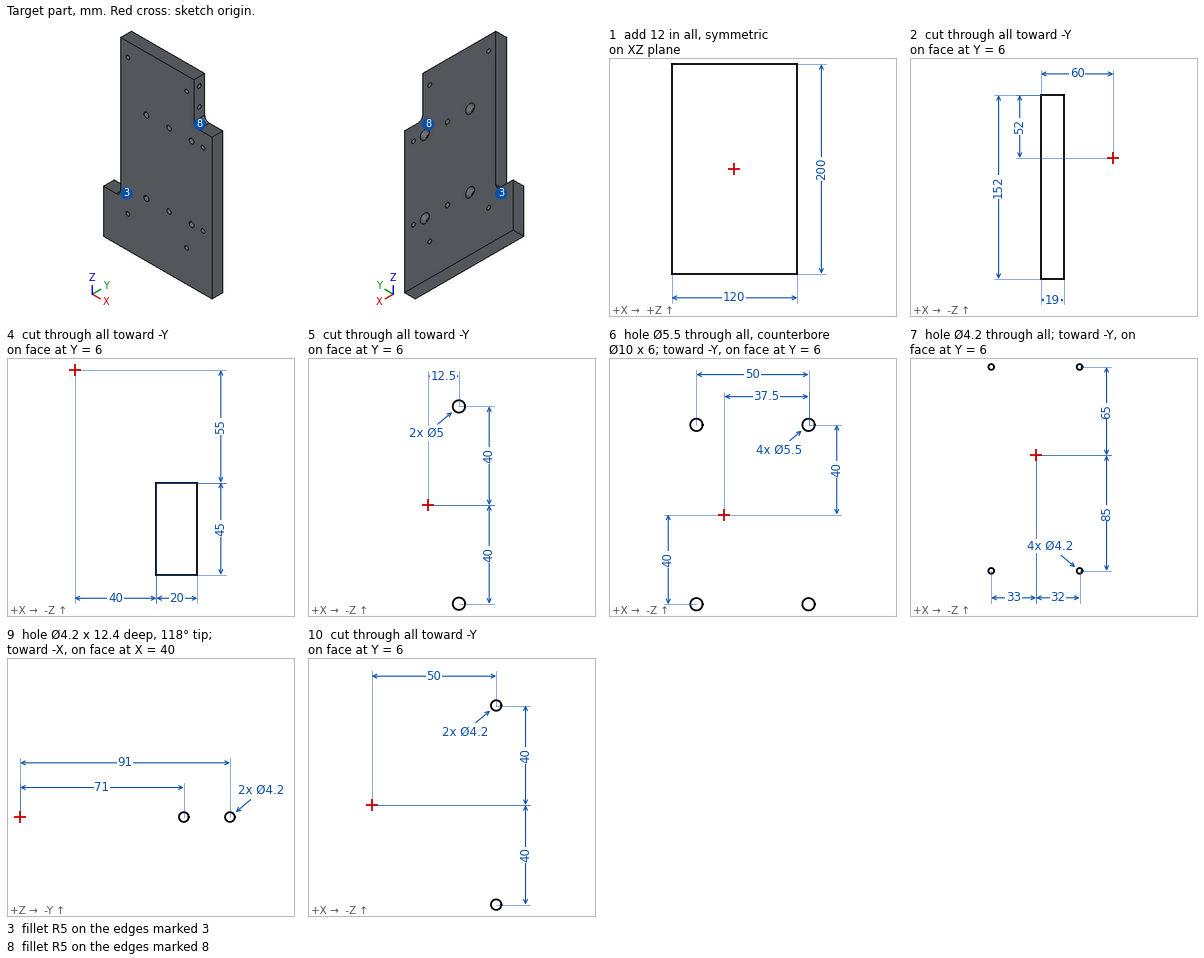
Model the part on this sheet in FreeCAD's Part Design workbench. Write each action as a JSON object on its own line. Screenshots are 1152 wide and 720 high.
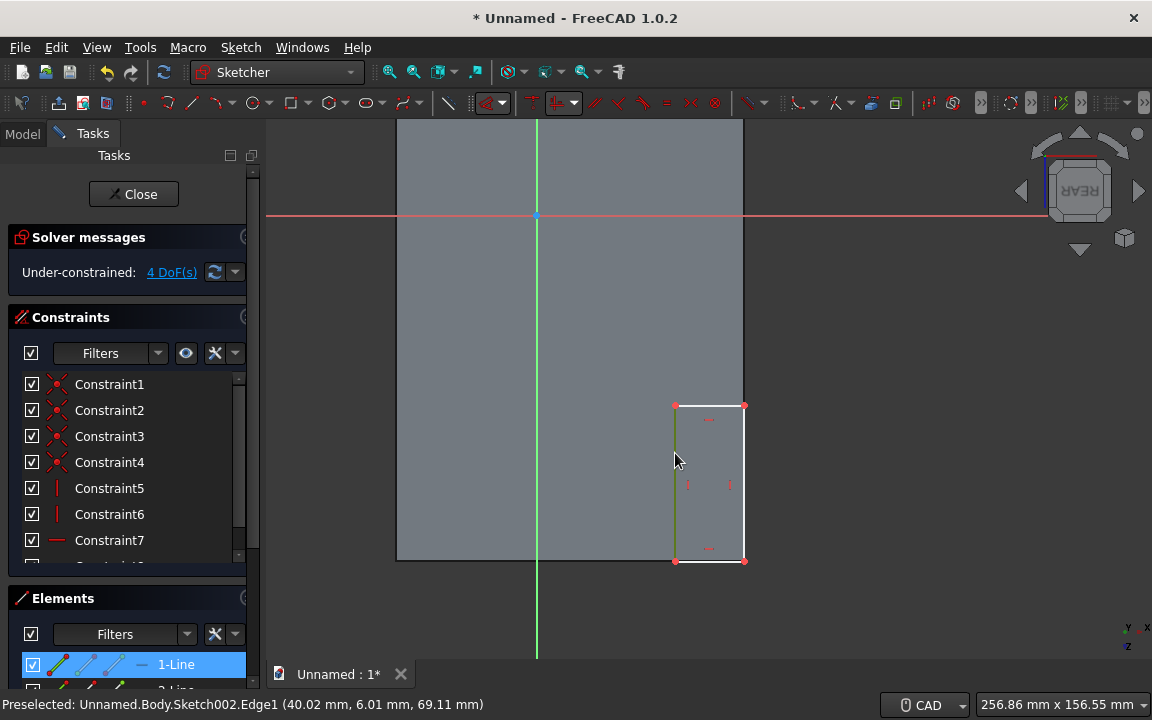
{"action": "left_click", "coordinate": [504, 104]}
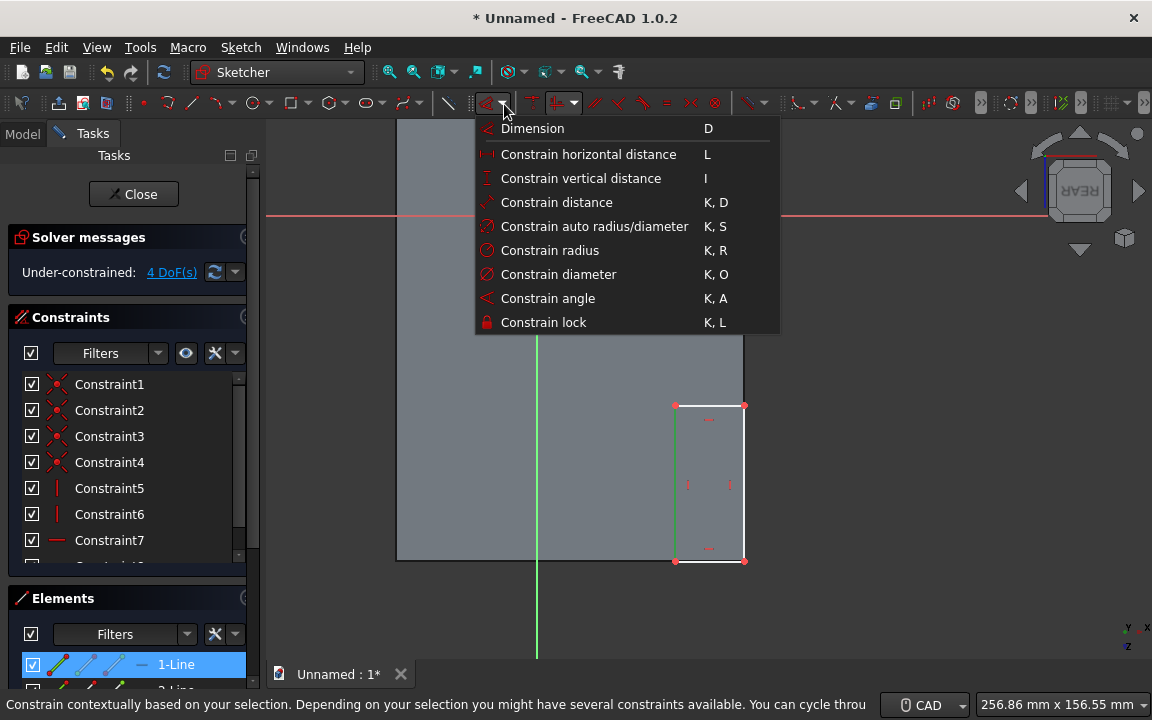
{"action": "left_click", "coordinate": [628, 178]}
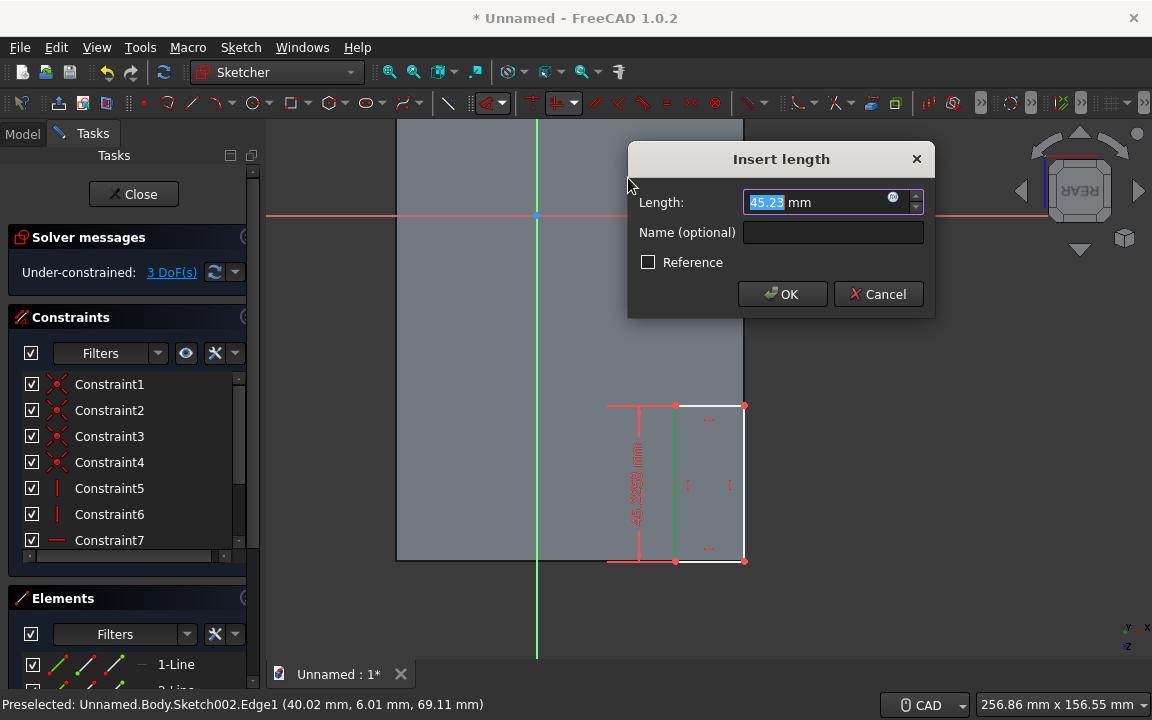
{"action": "type", "text": "45"}
{"action": "key", "text": "Return"}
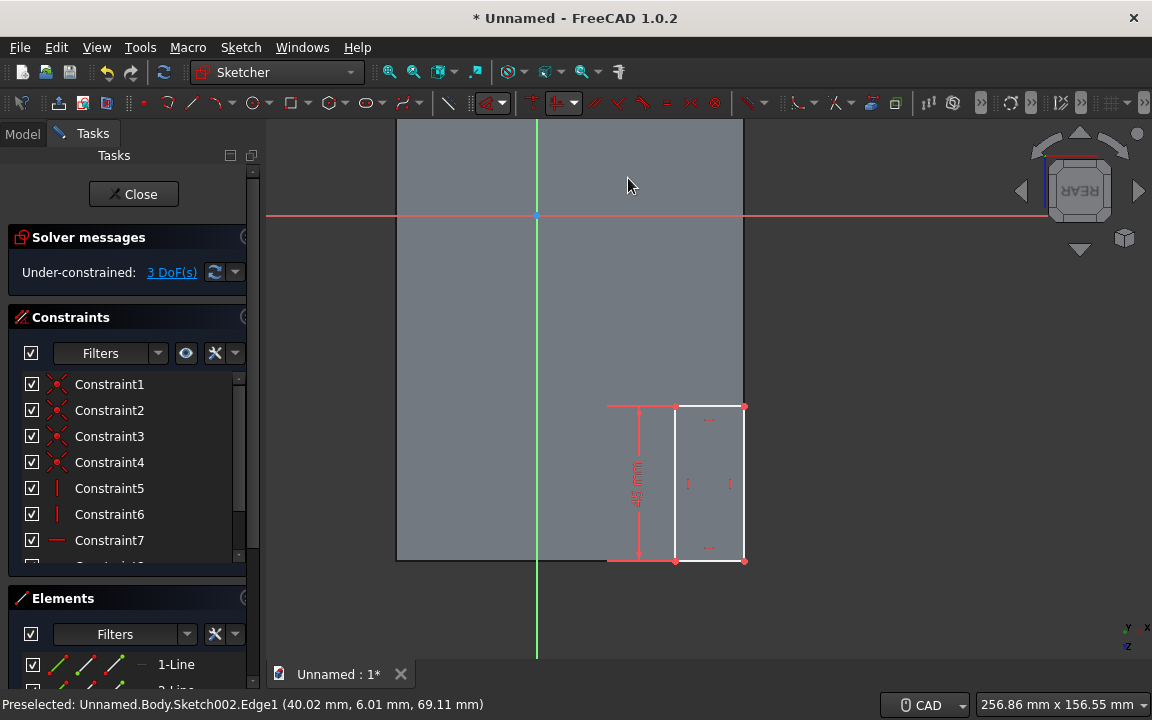
{"action": "left_click", "coordinate": [696, 561]}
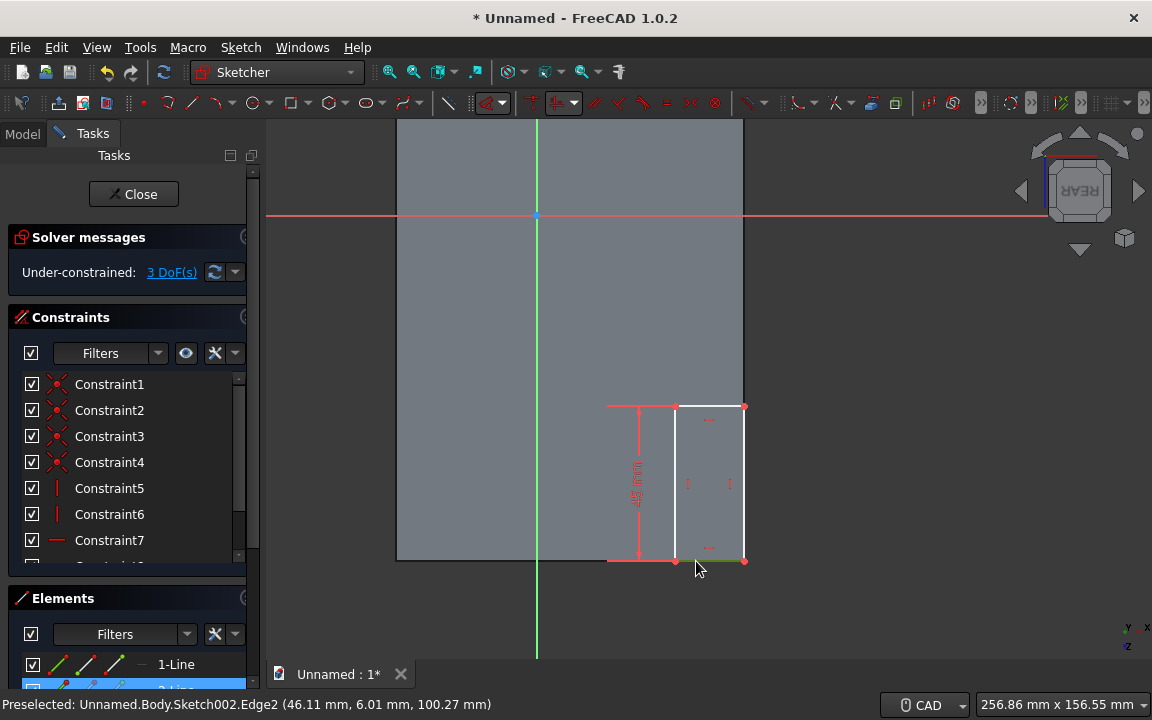
{"action": "left_click", "coordinate": [504, 104]}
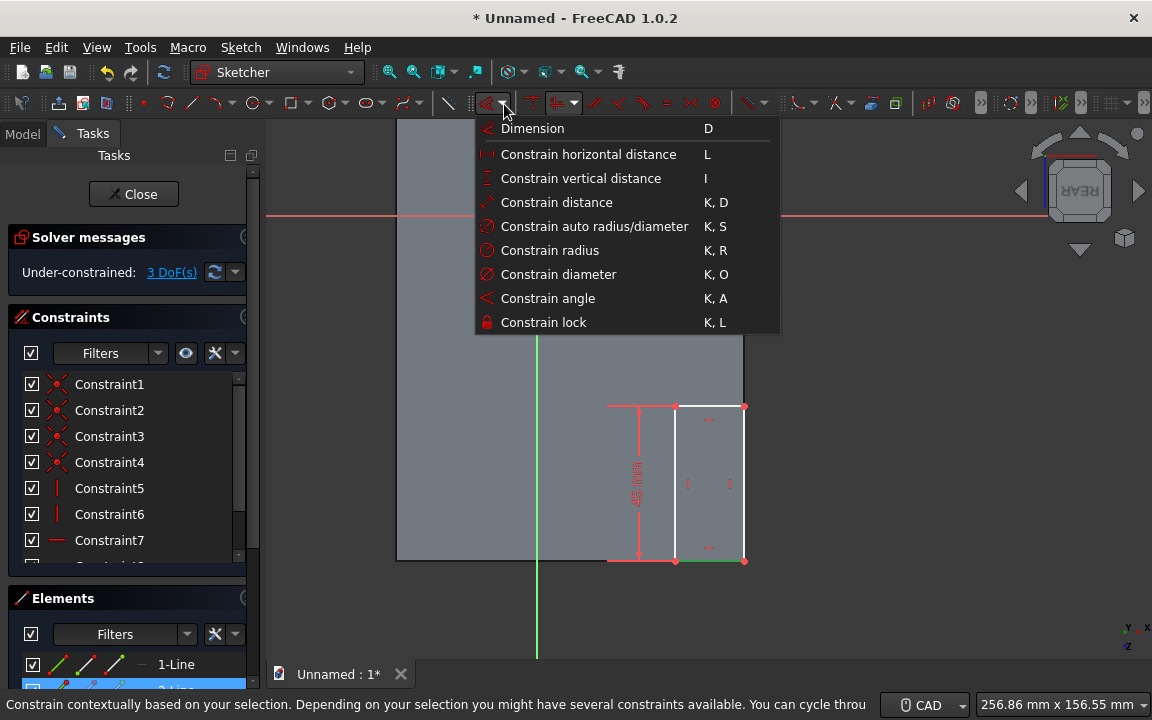
{"action": "left_click", "coordinate": [628, 154]}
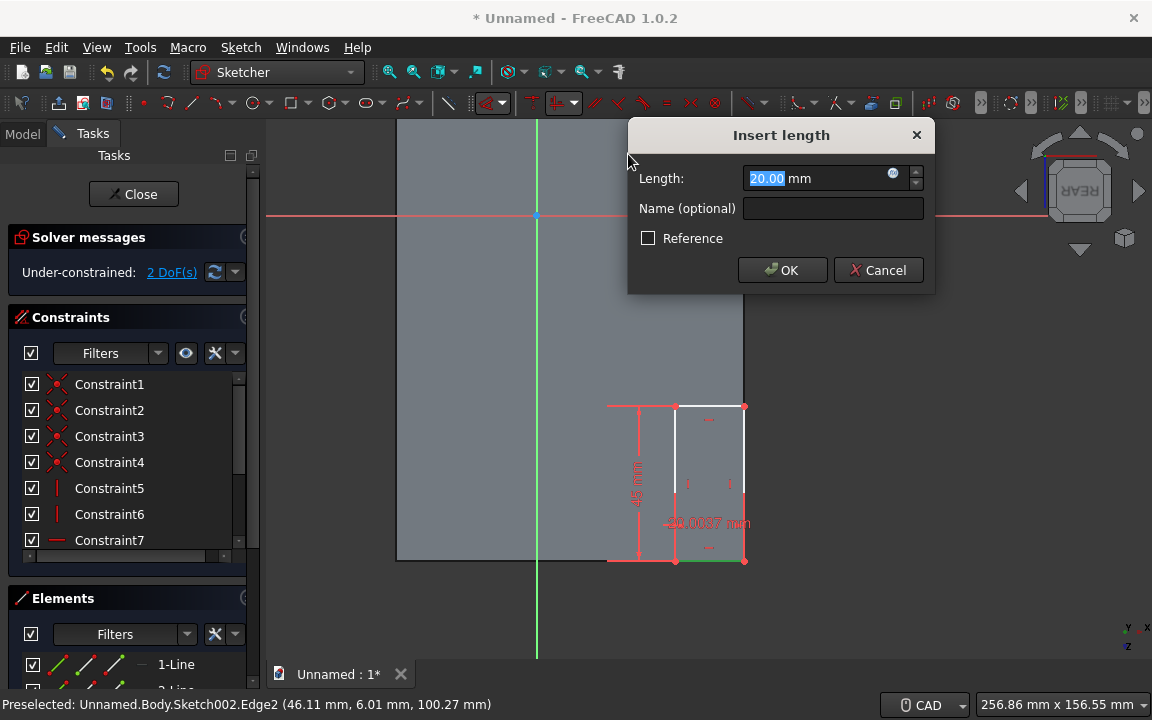
{"action": "type", "text": "20"}
{"action": "key", "text": "Return"}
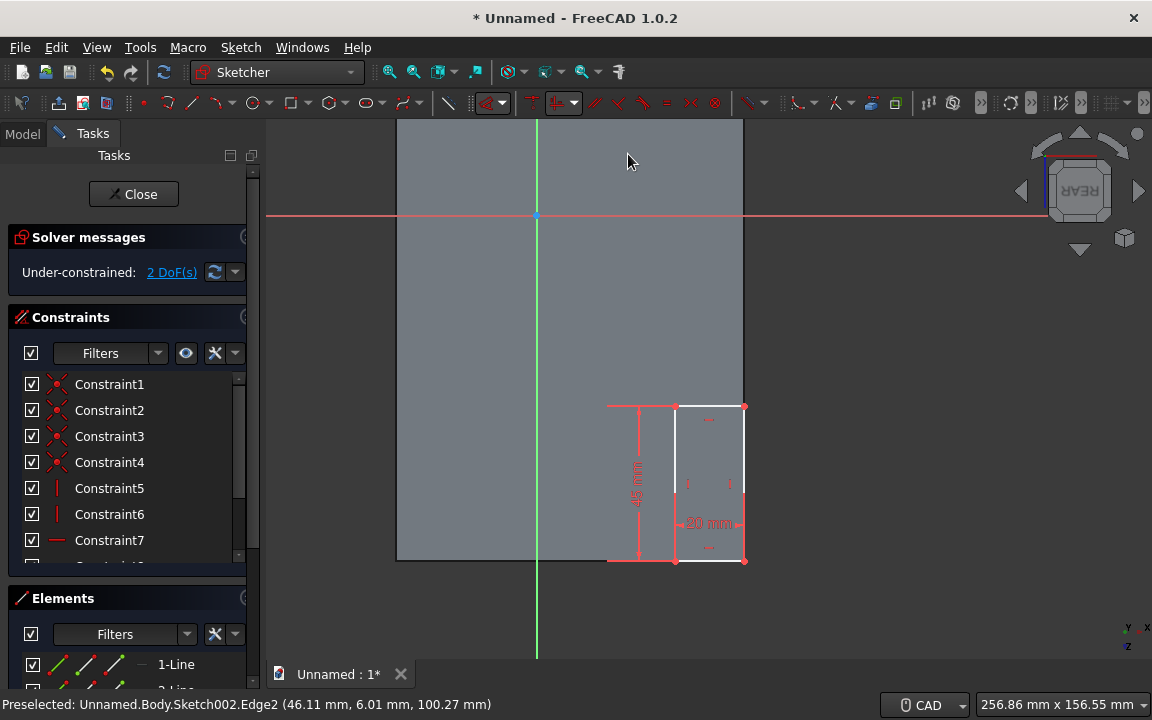
{"action": "left_click", "coordinate": [675, 406]}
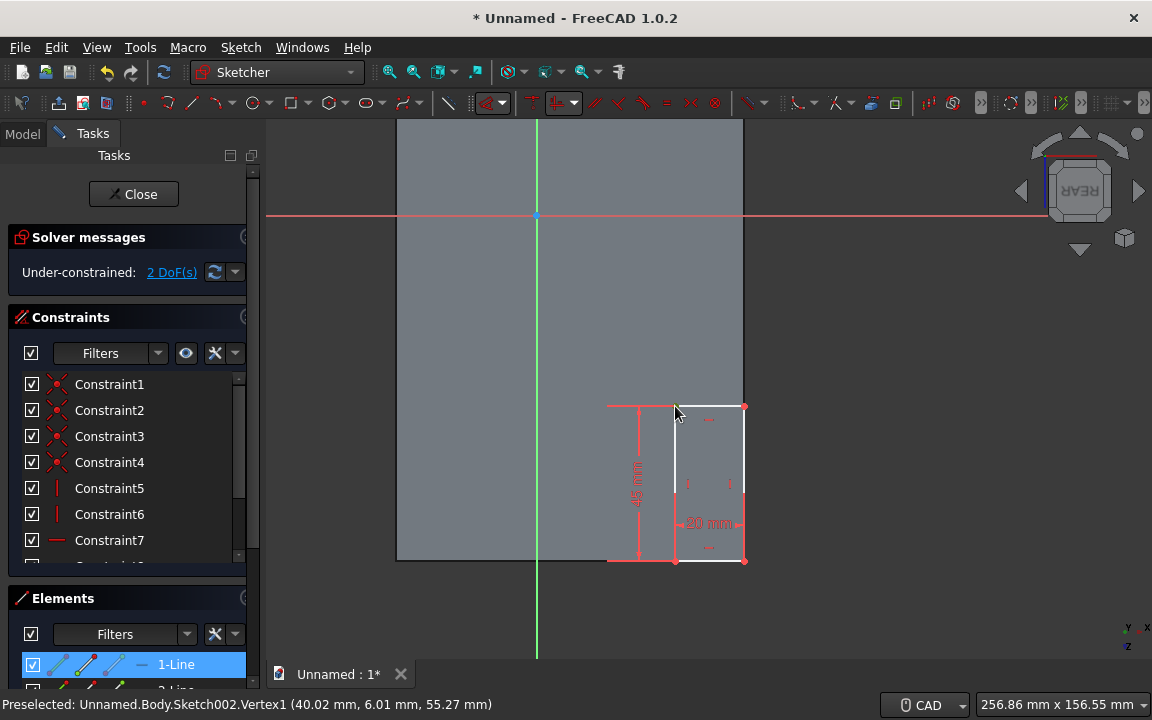
{"action": "key", "text": "l"}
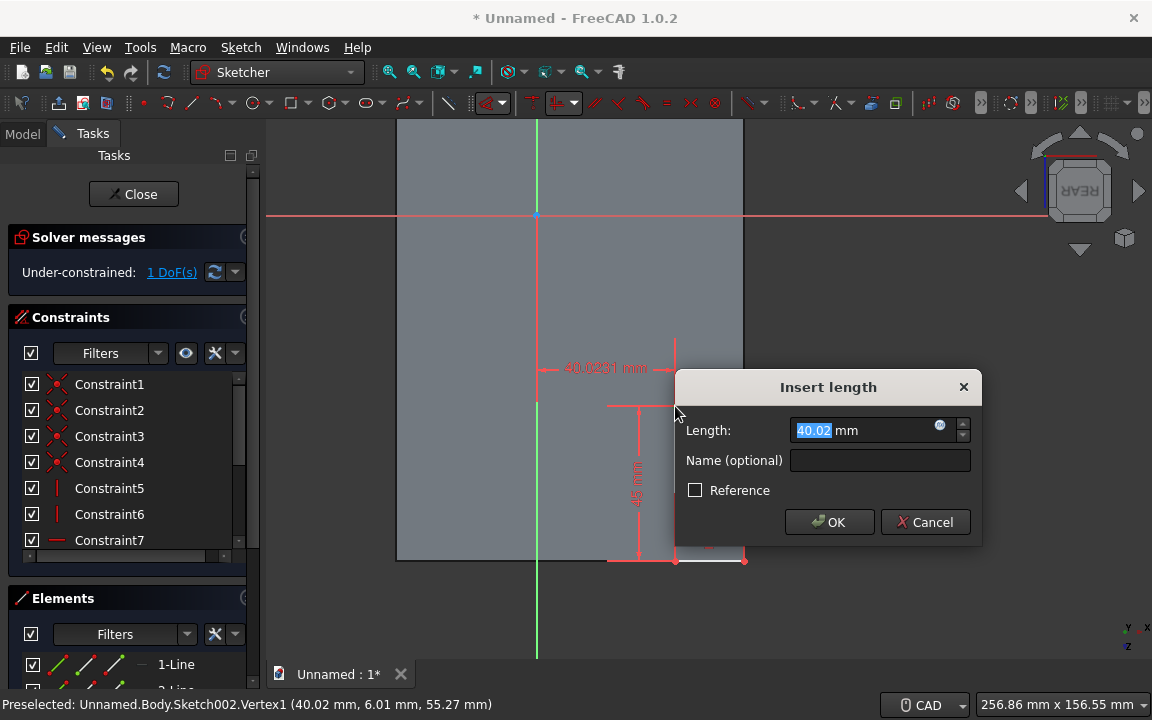
{"action": "type", "text": "40"}
{"action": "key", "text": "Return"}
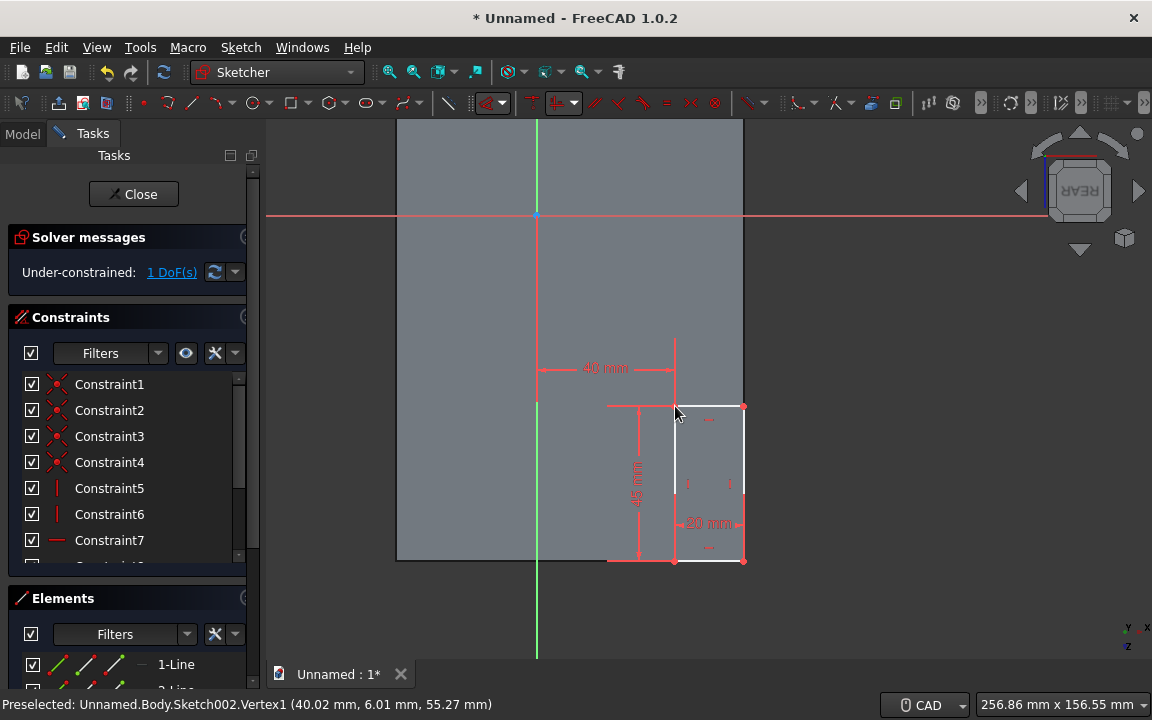
{"action": "left_click", "coordinate": [675, 406]}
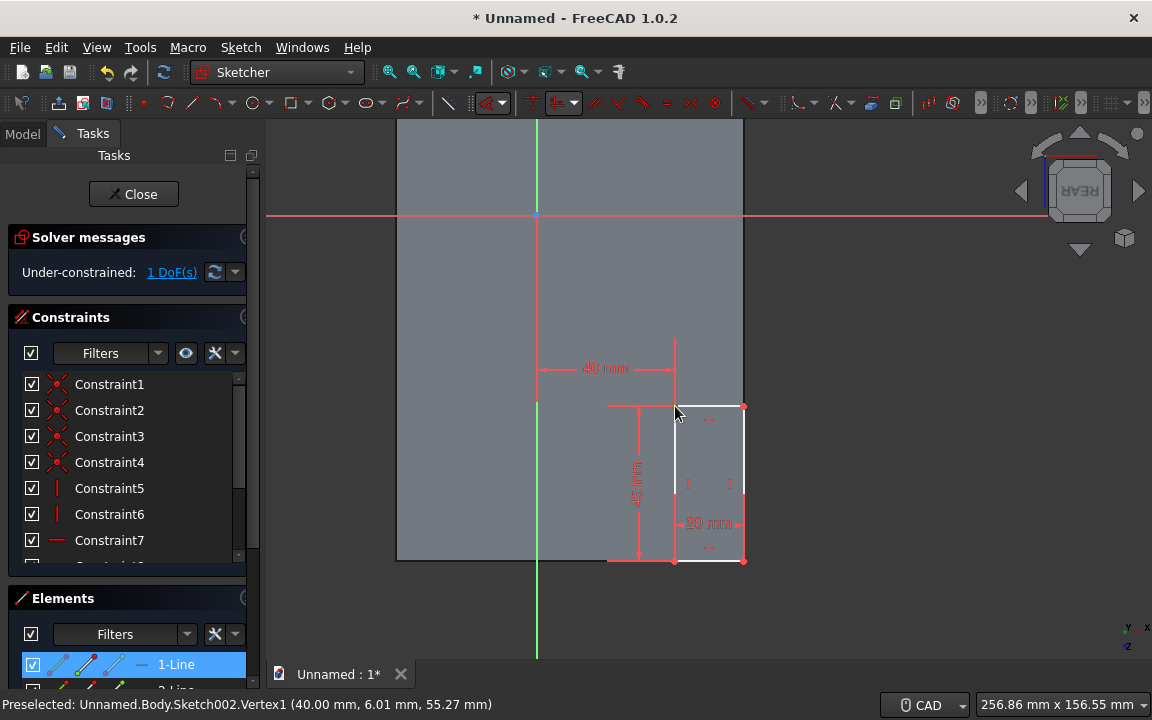
{"action": "key", "text": "i"}